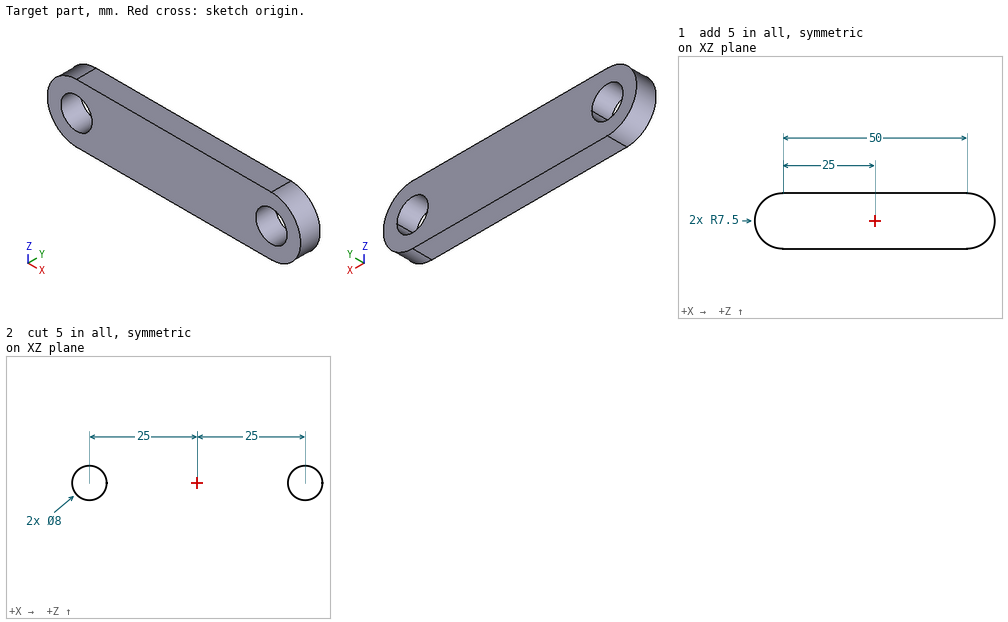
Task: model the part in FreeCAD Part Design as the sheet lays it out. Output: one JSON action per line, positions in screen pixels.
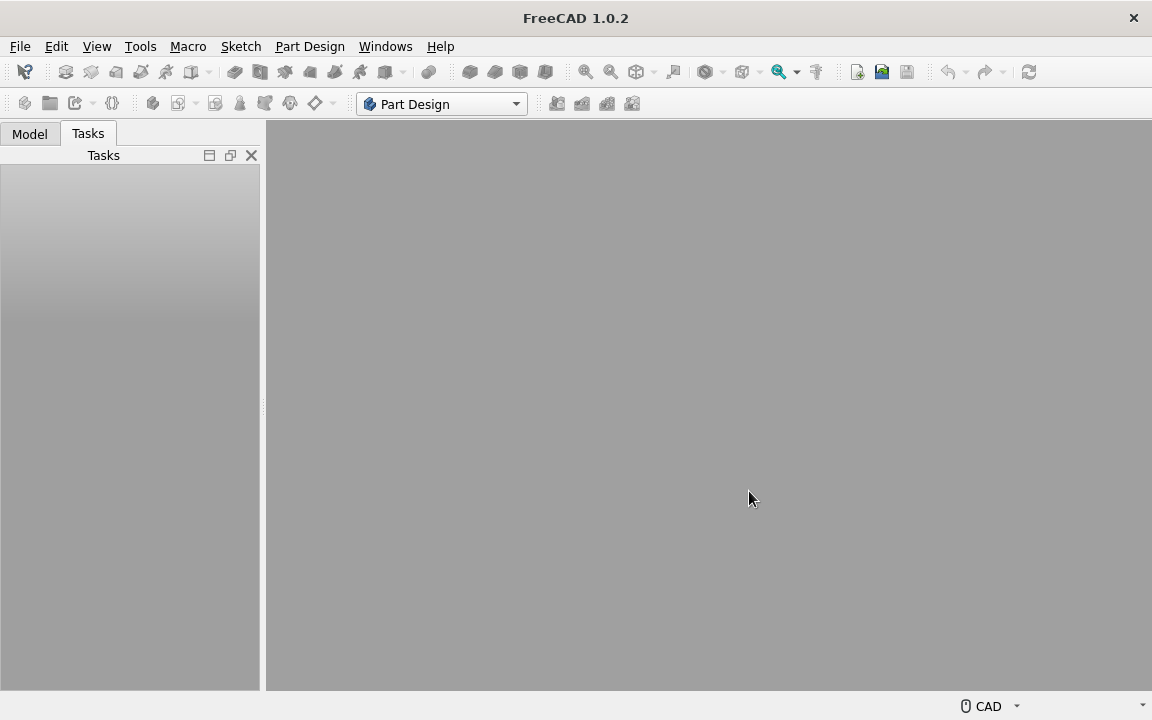
{"action": "left_click", "coordinate": [857, 72]}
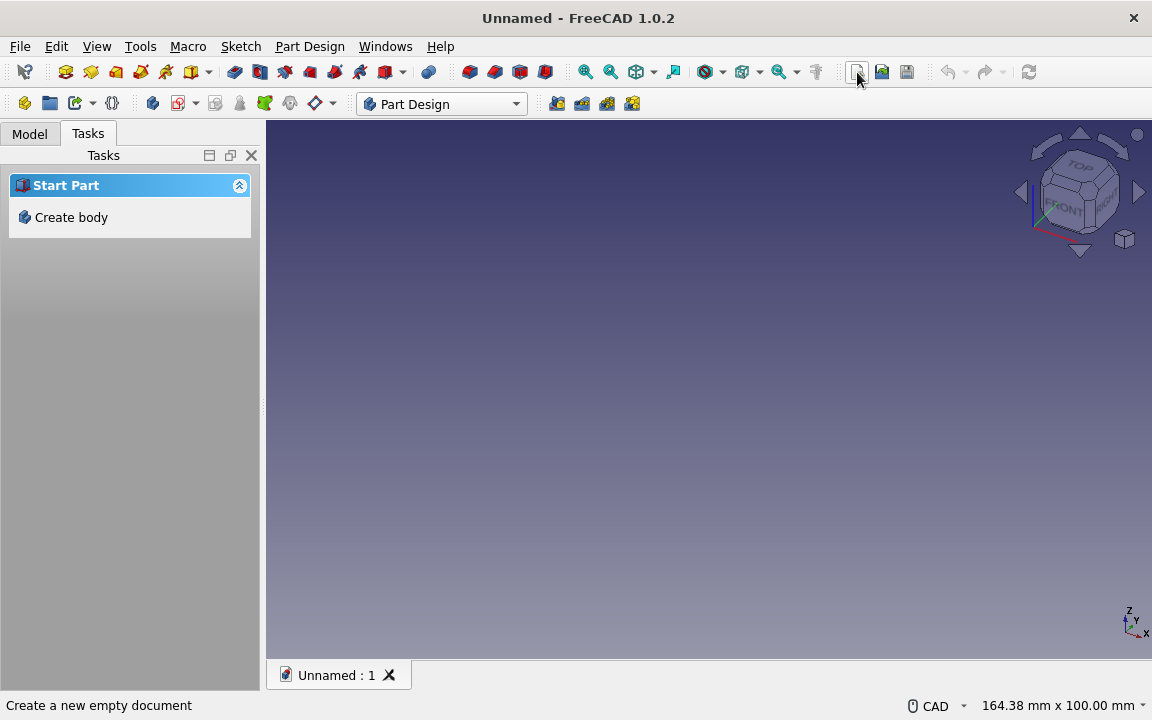
{"action": "left_click", "coordinate": [178, 104]}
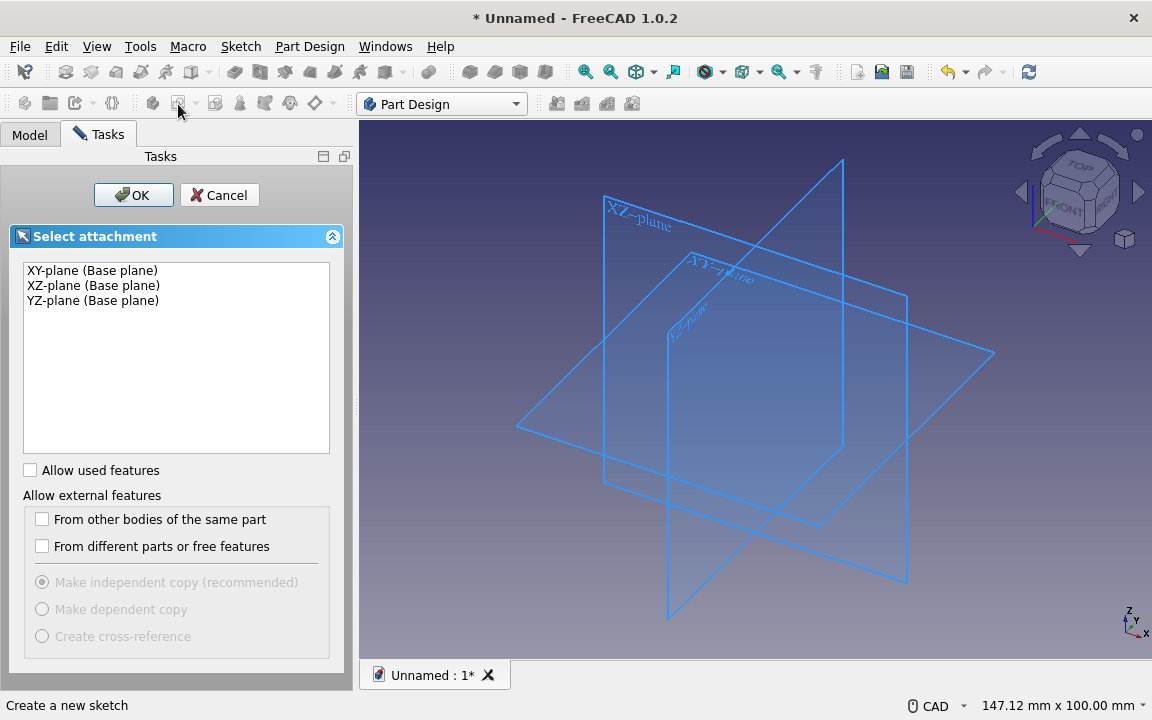
{"action": "left_click", "coordinate": [84, 286]}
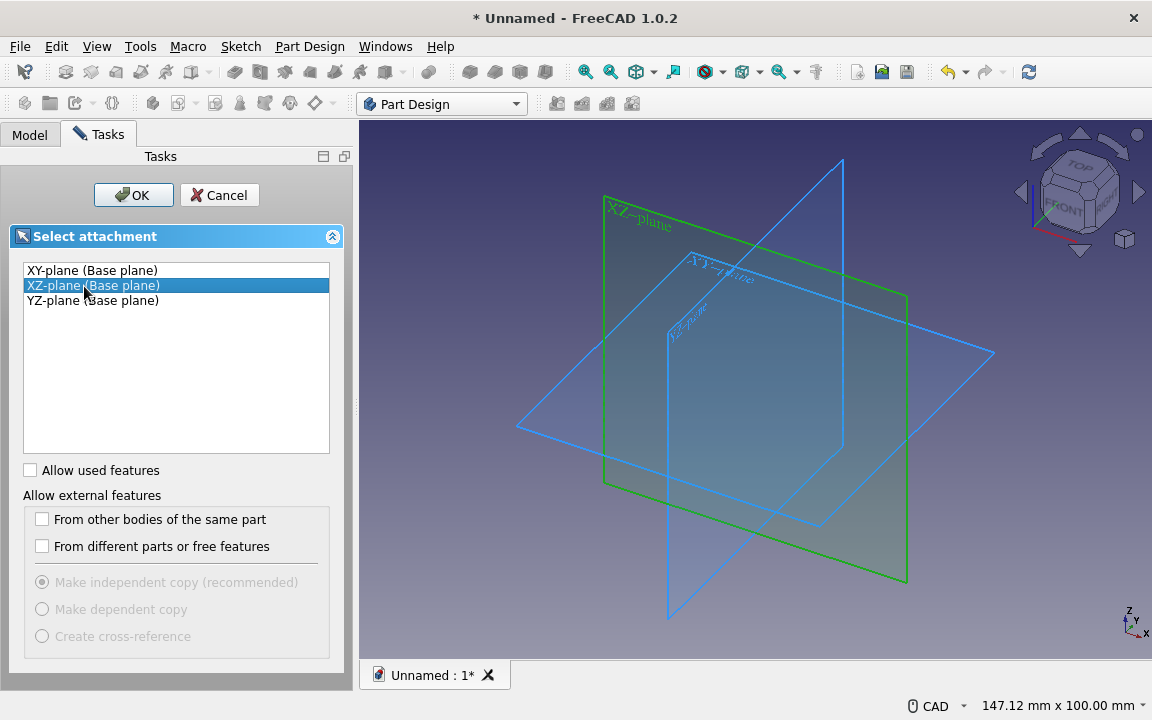
{"action": "left_click", "coordinate": [134, 195]}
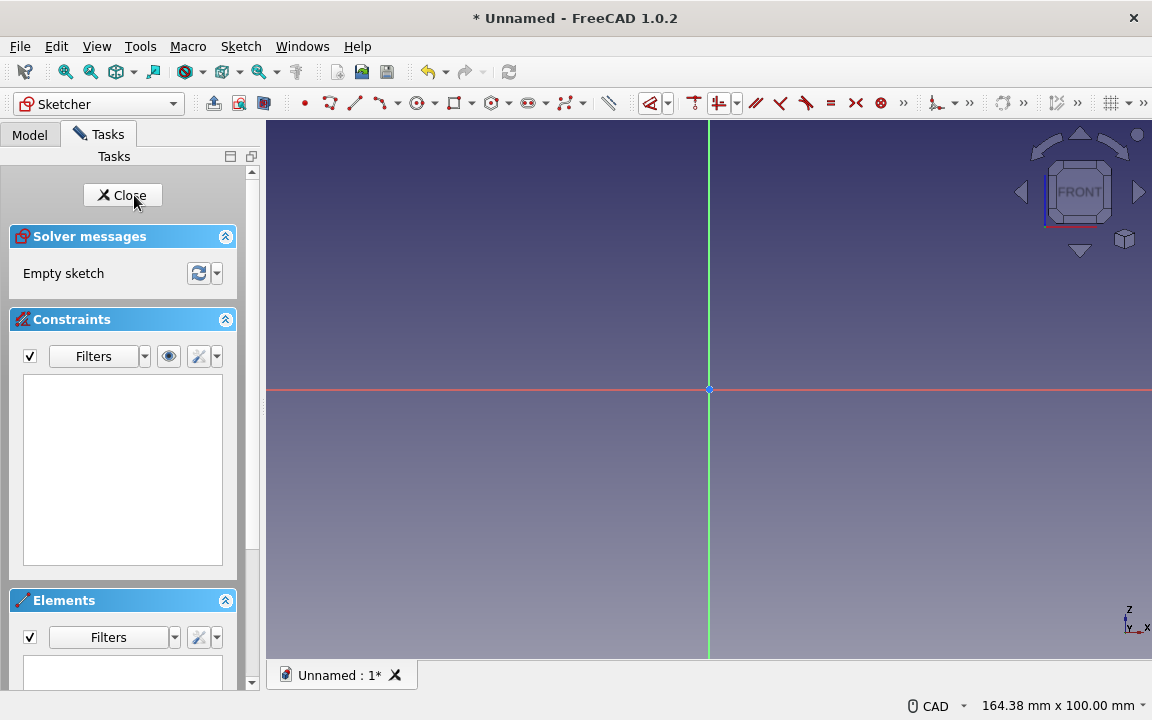
{"action": "scroll", "coordinate": [848, 390], "scroll_direction": "up", "scroll_amount": 2}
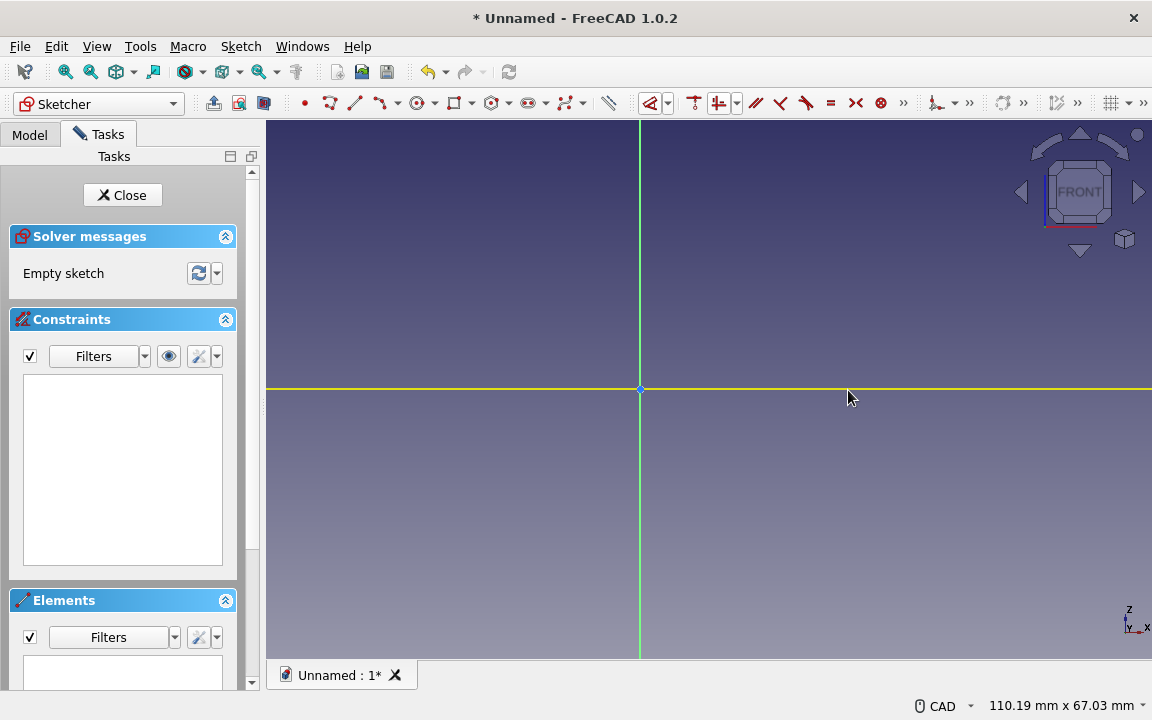
{"action": "left_click", "coordinate": [528, 104]}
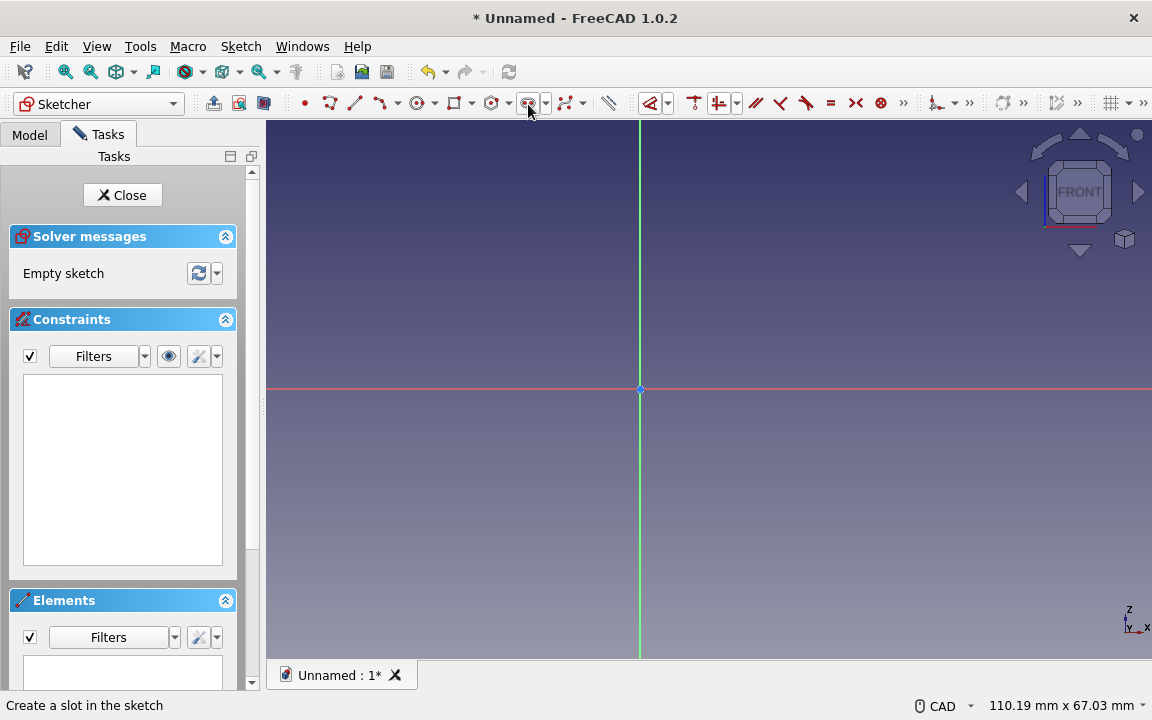
{"action": "left_click", "coordinate": [439, 389]}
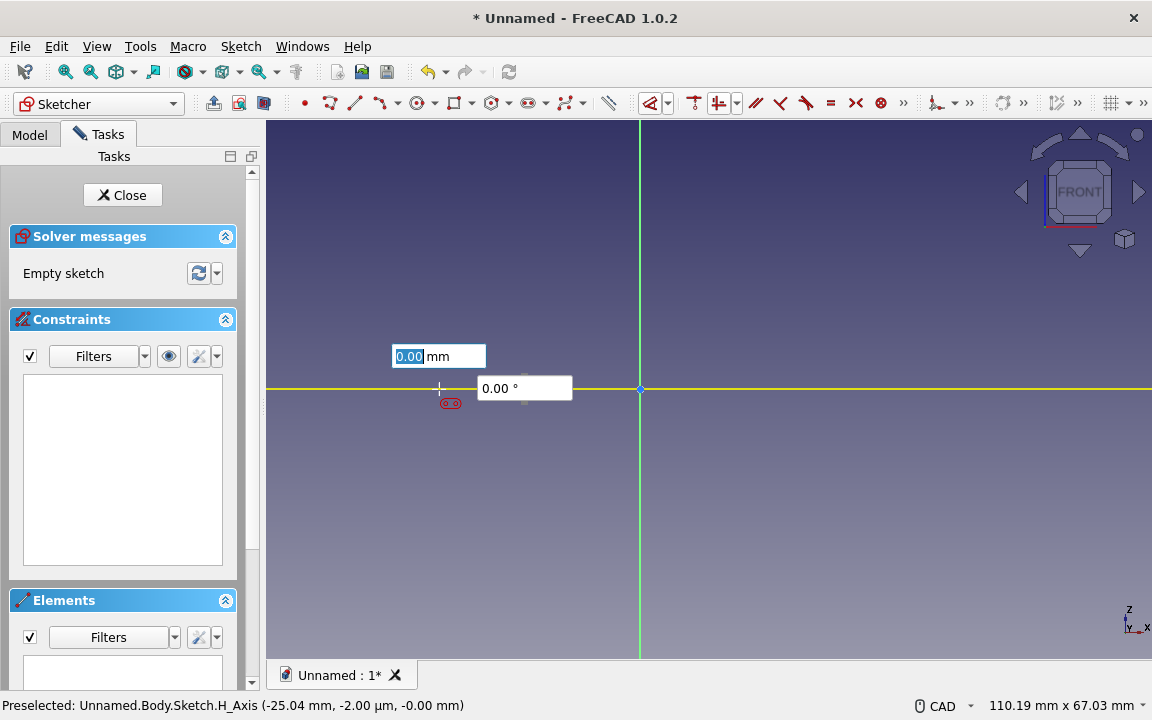
{"action": "left_click", "coordinate": [841, 380]}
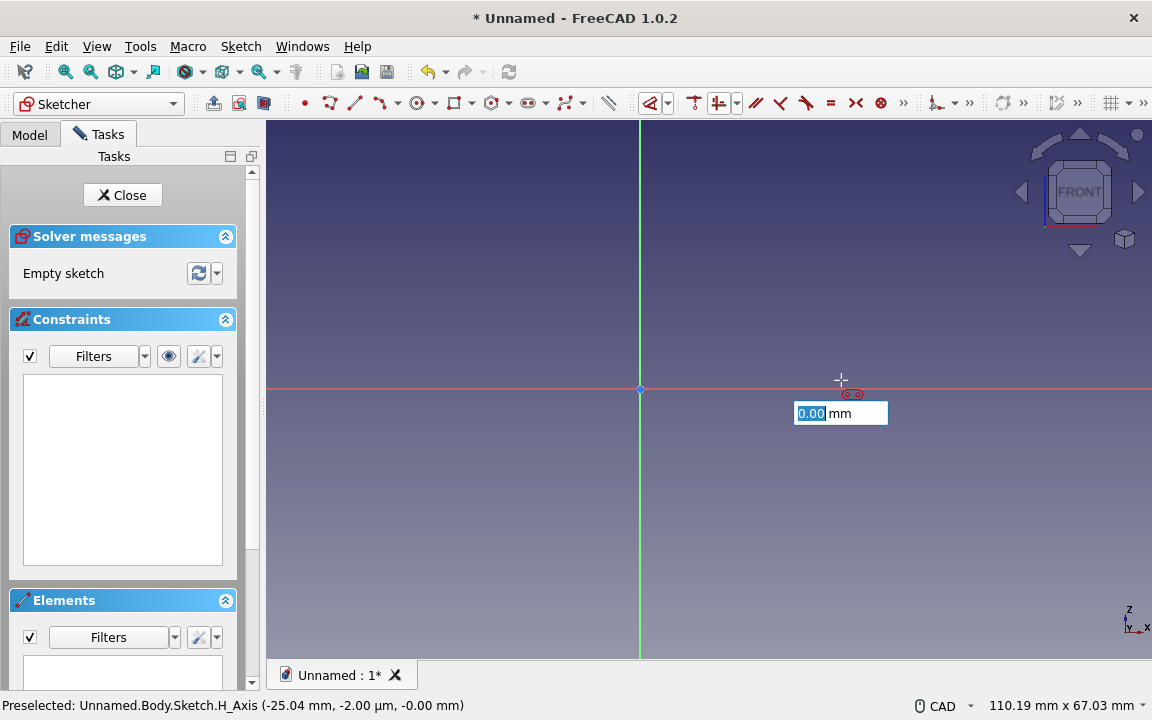
{"action": "left_click", "coordinate": [701, 449]}
{"action": "key", "text": "Escape"}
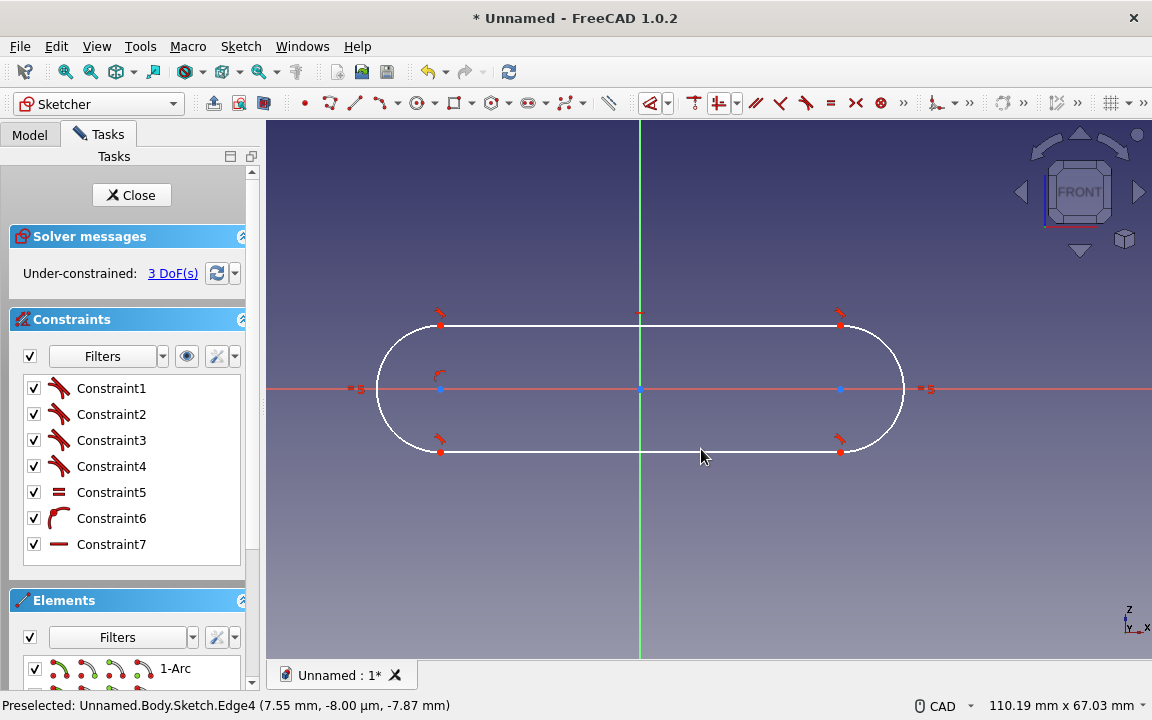
{"action": "left_click", "coordinate": [650, 104]}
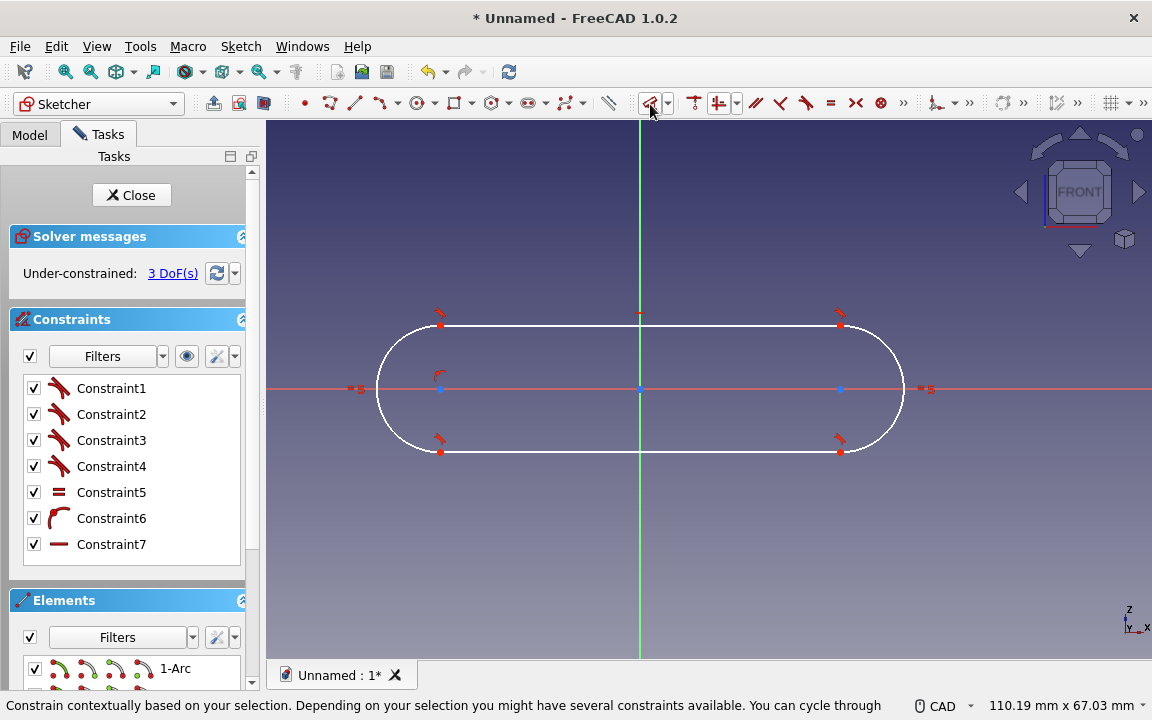
{"action": "left_click", "coordinate": [389, 352]}
{"action": "left_click", "coordinate": [363, 333]}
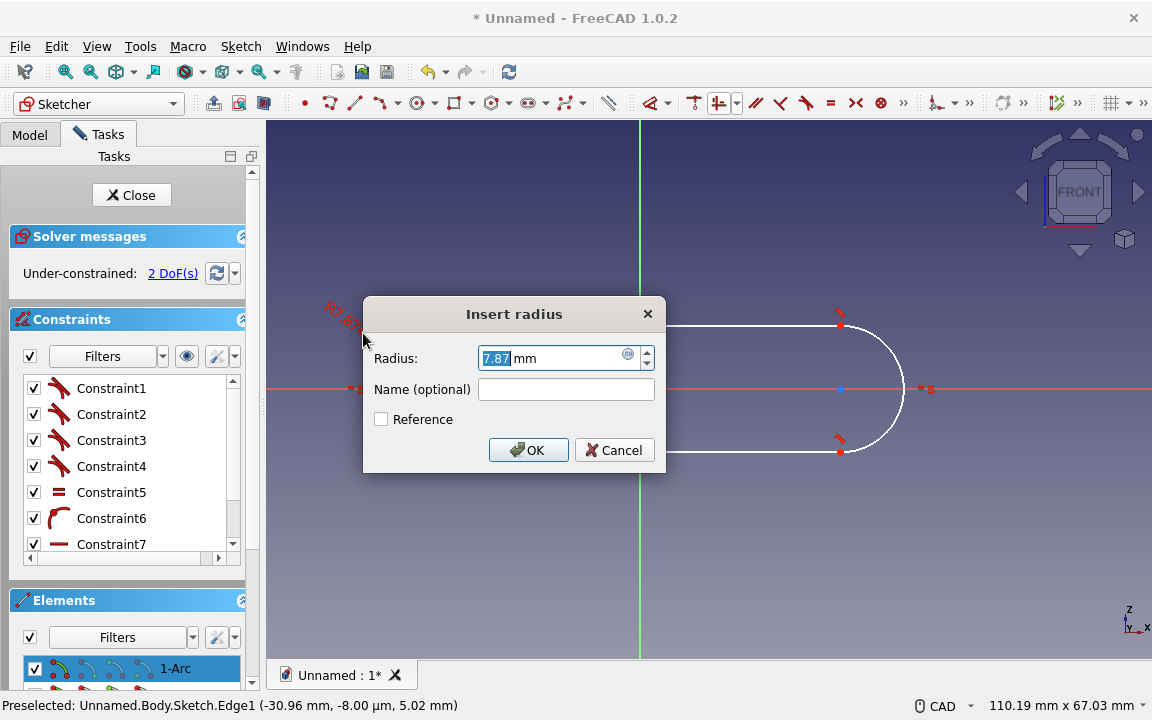
{"action": "type", "text": "7.5"}
{"action": "key", "text": "Return"}